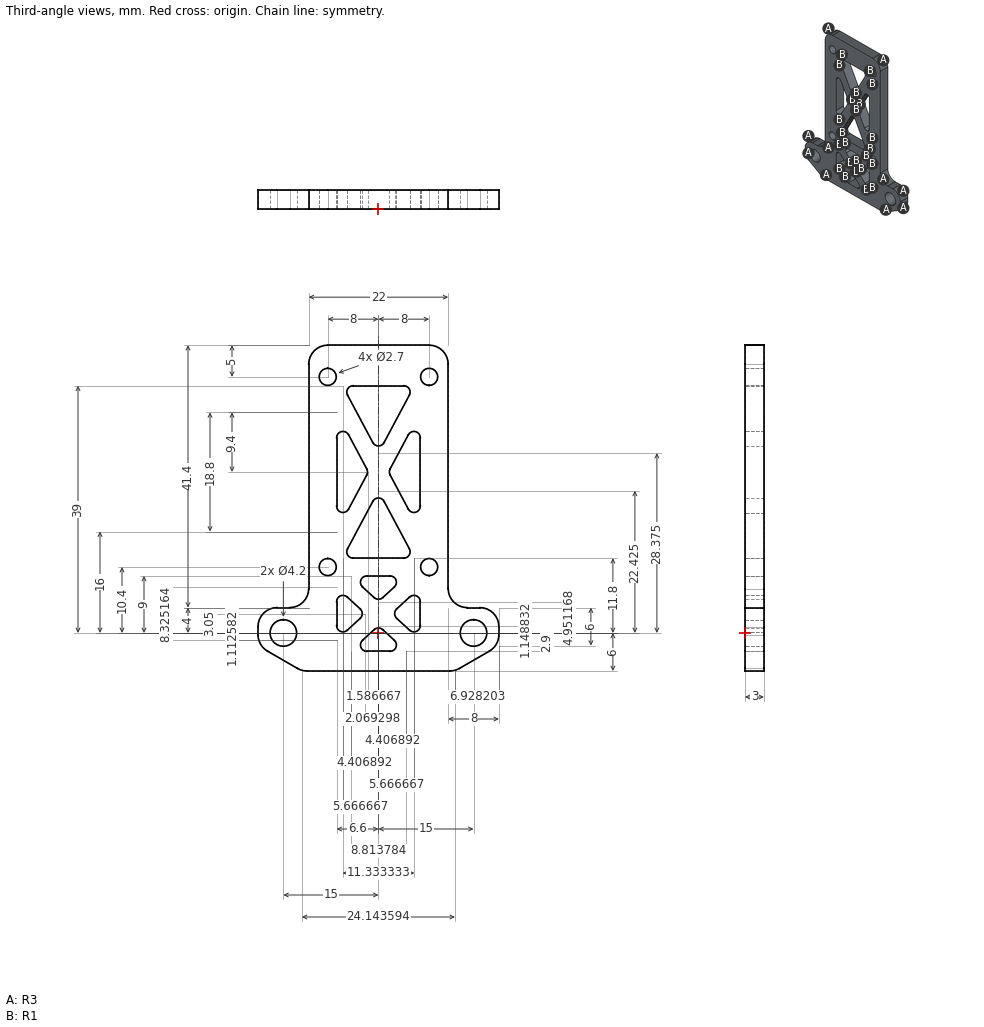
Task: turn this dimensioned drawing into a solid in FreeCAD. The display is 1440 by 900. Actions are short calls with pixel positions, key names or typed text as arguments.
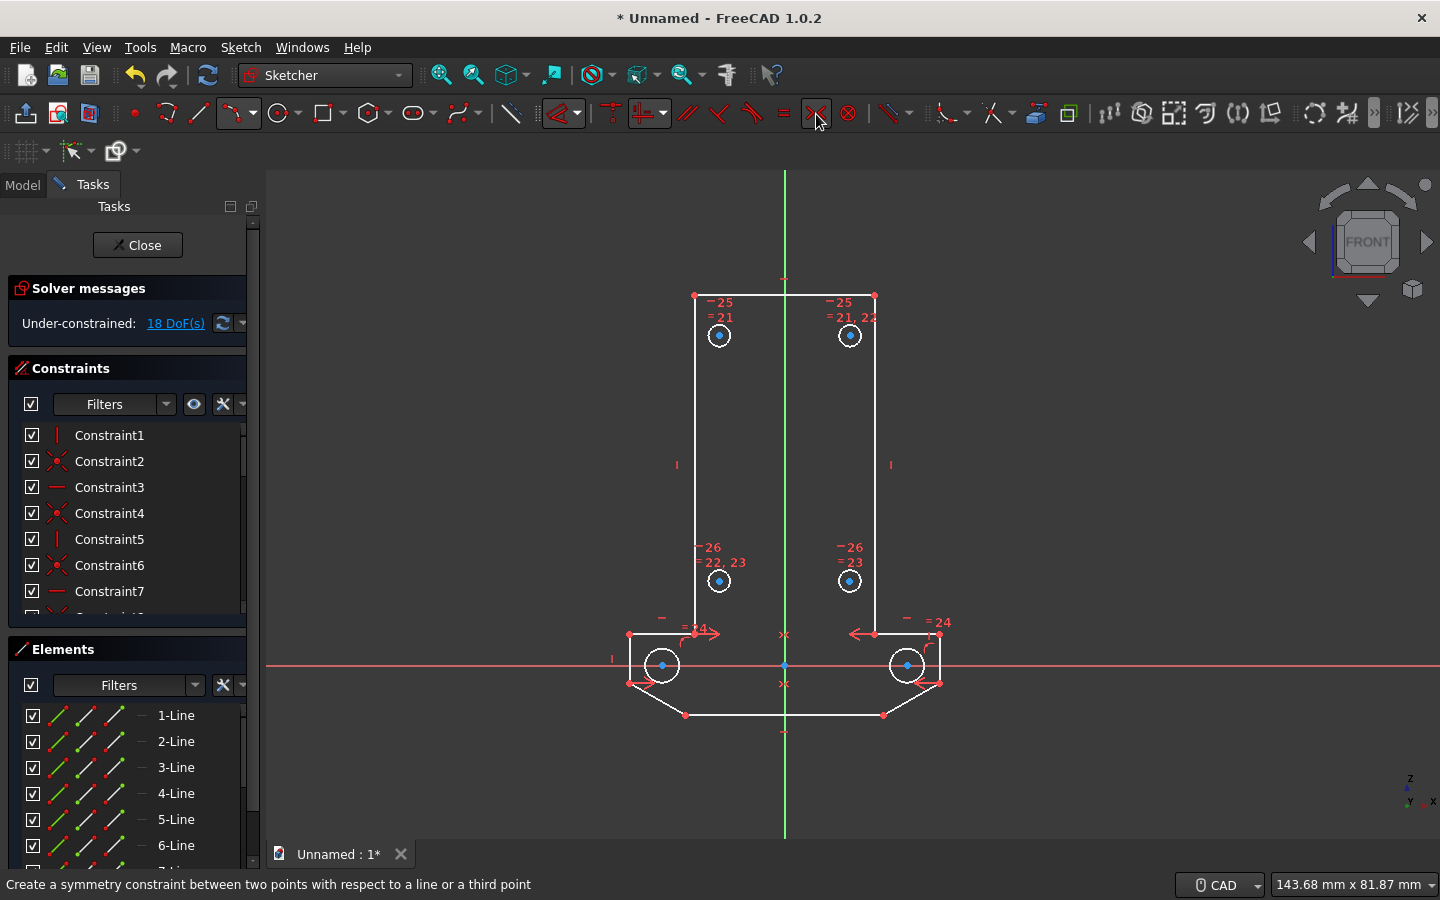
scroll(727, 328, up, 3)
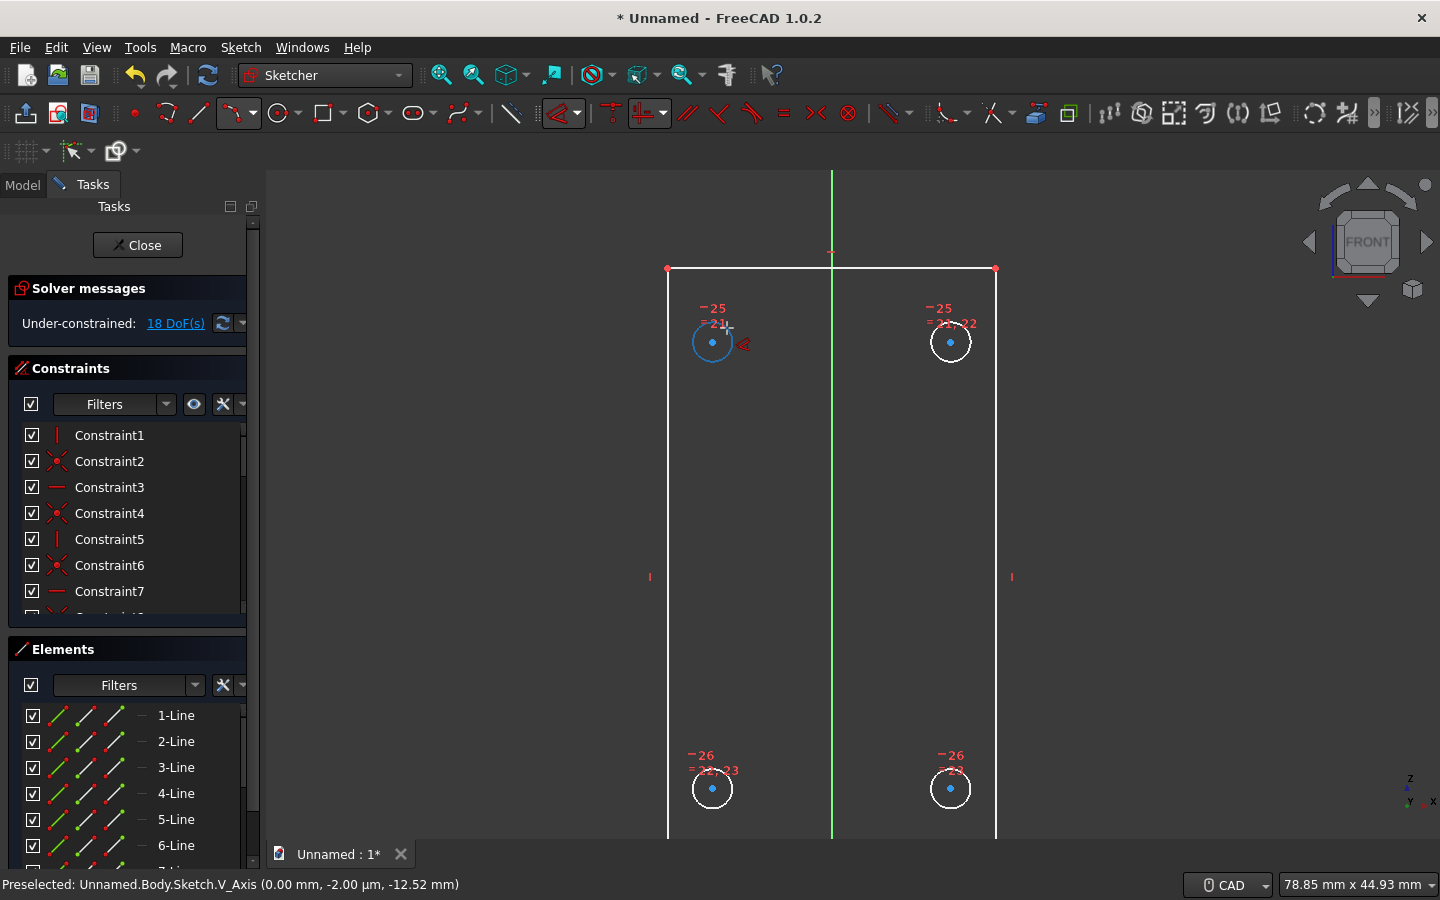
click(727, 328)
click(750, 306)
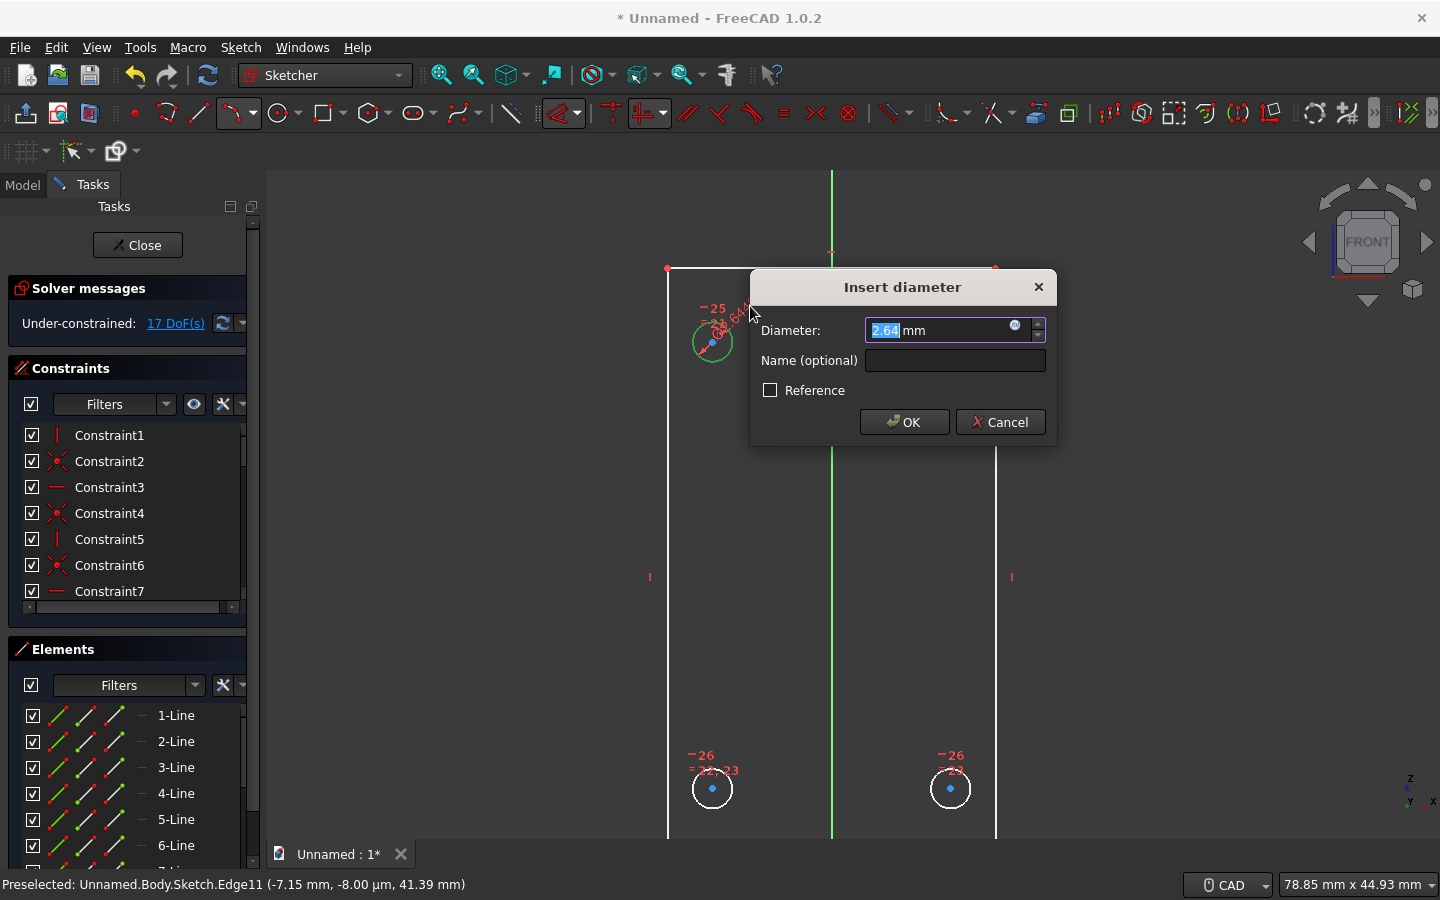
text(2.7)
key(Return)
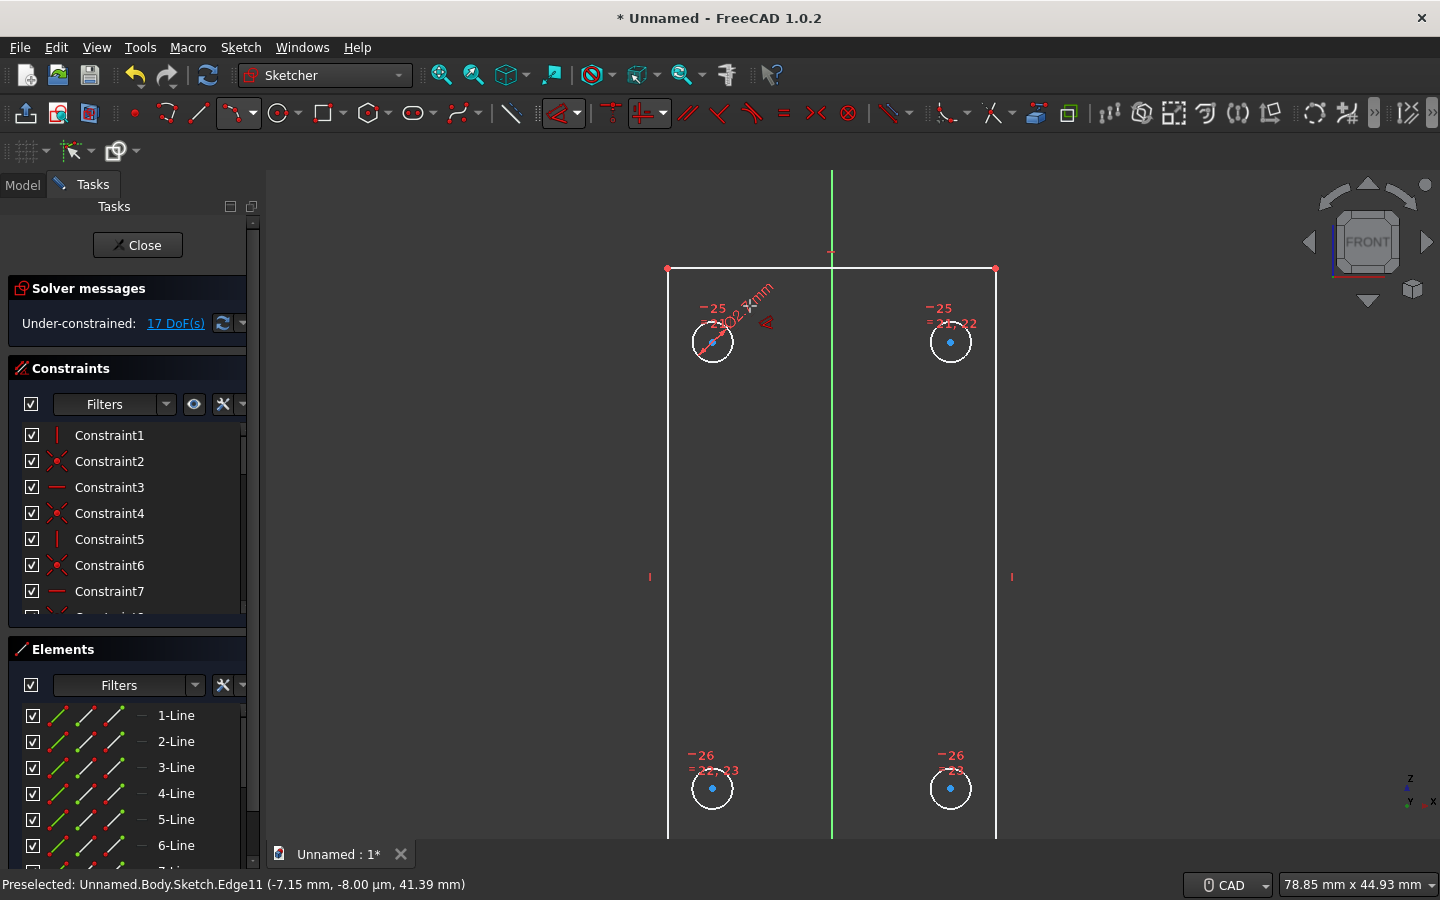
scroll(727, 328, down, 3)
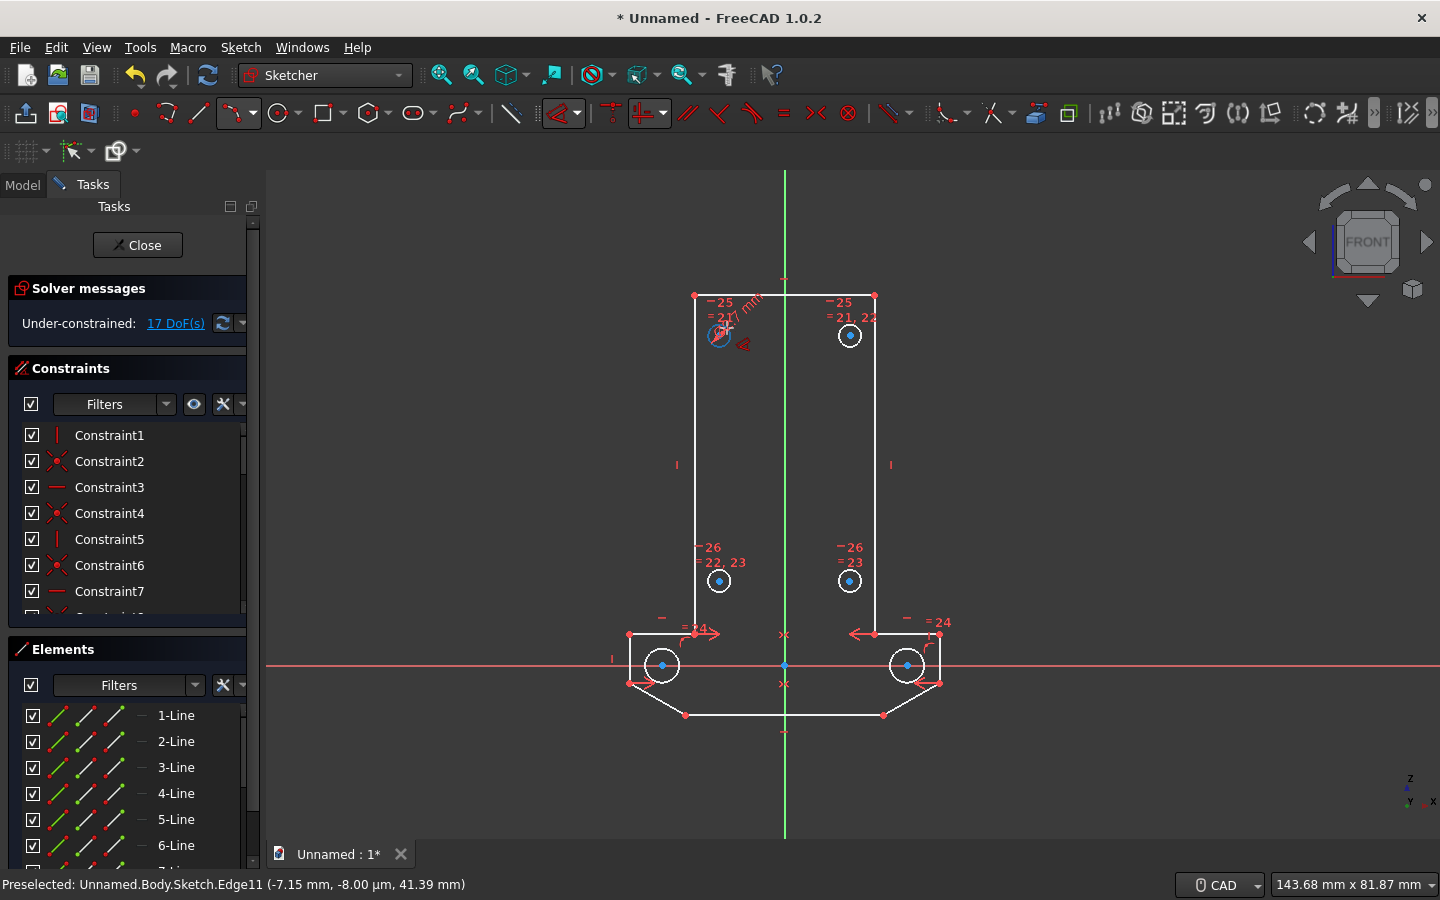
click(674, 654)
click(709, 652)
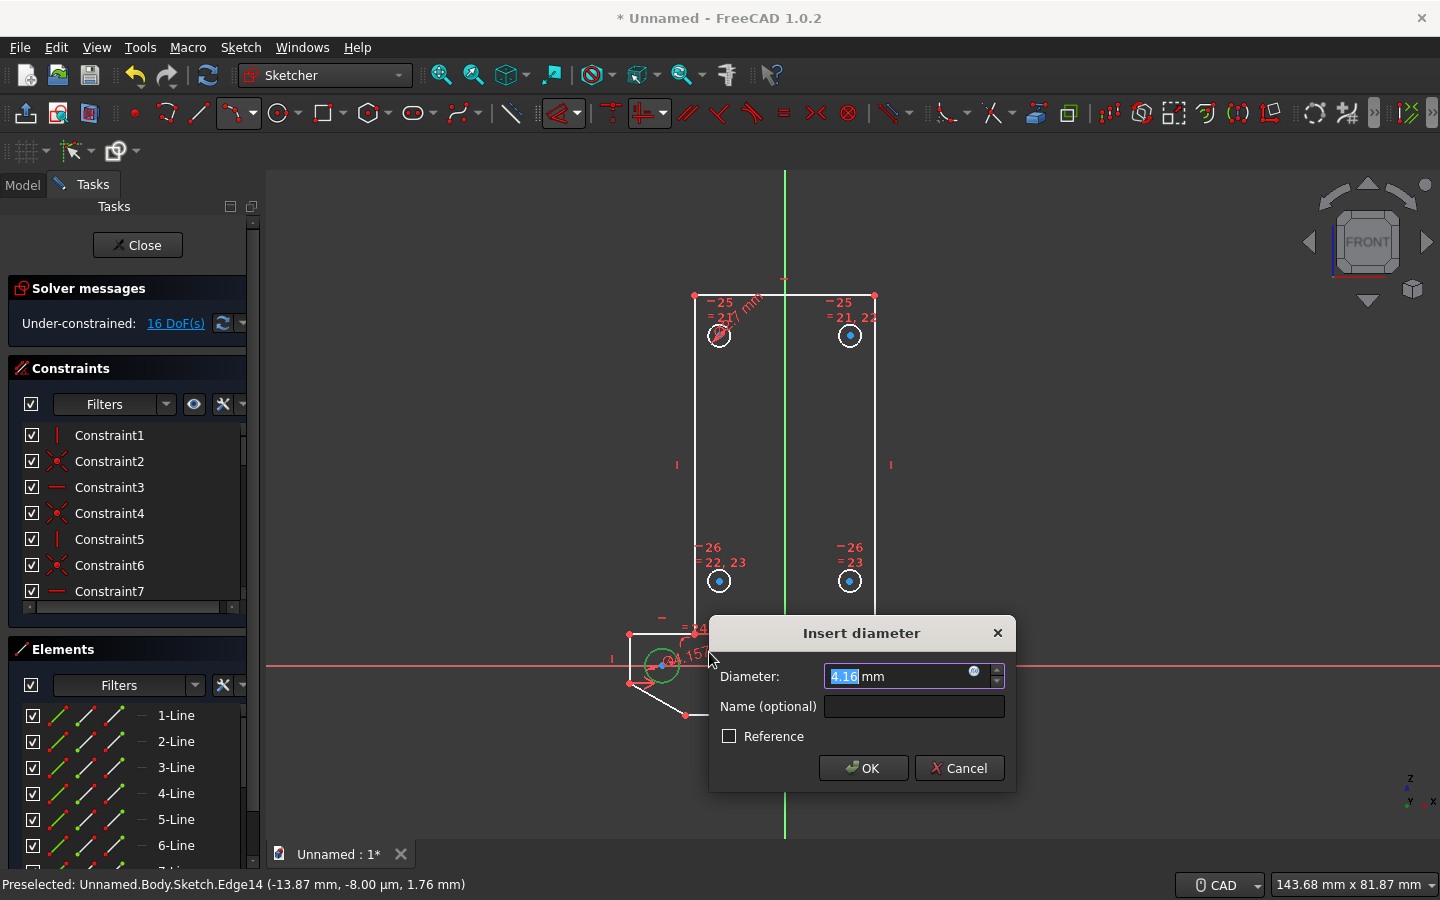
text(4.2)
key(Return)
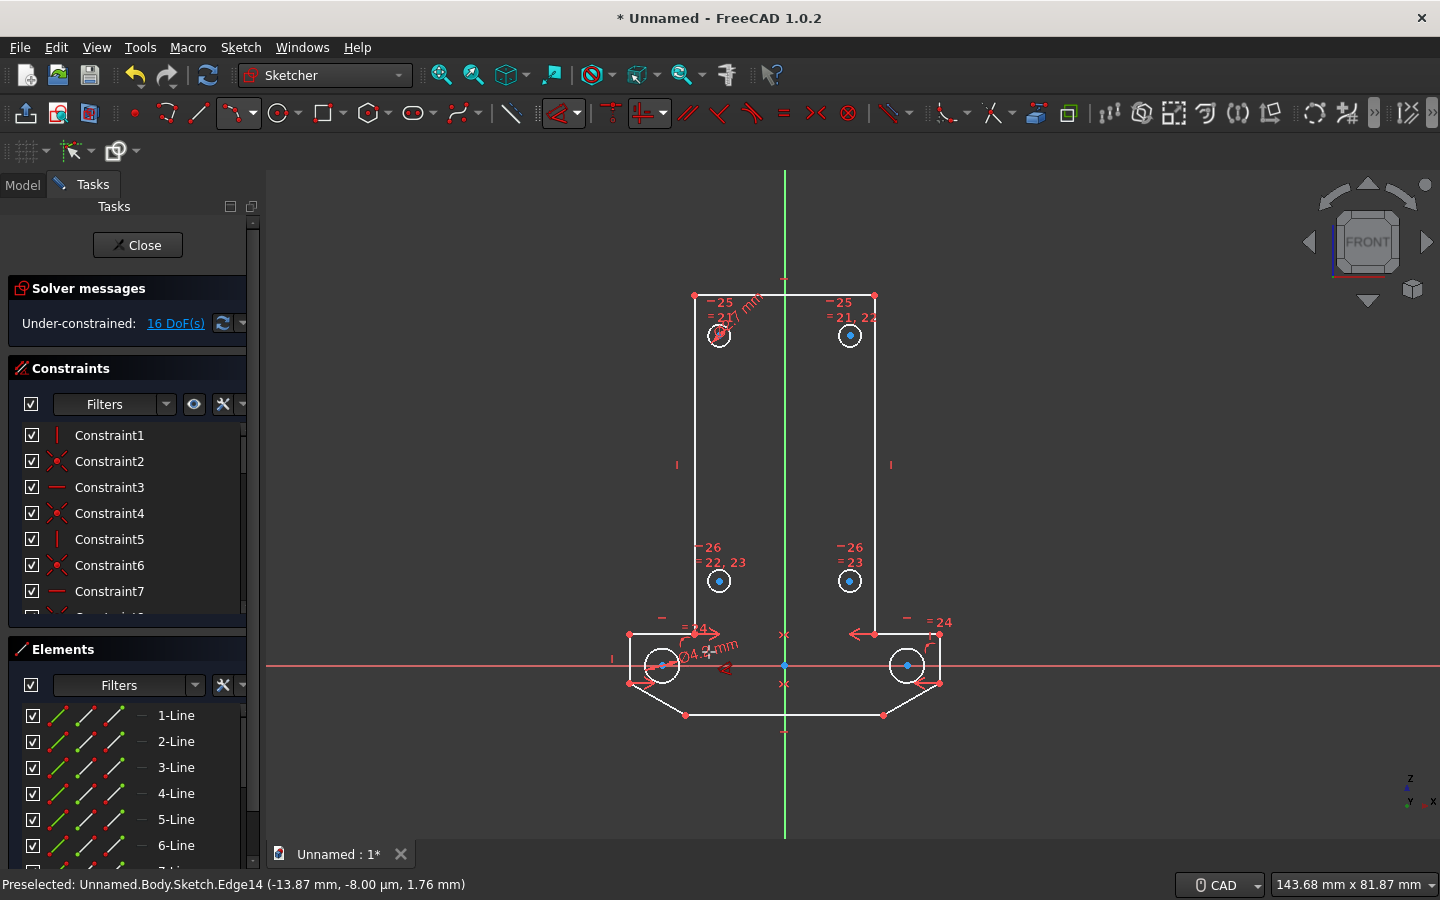
click(894, 634)
click(907, 600)